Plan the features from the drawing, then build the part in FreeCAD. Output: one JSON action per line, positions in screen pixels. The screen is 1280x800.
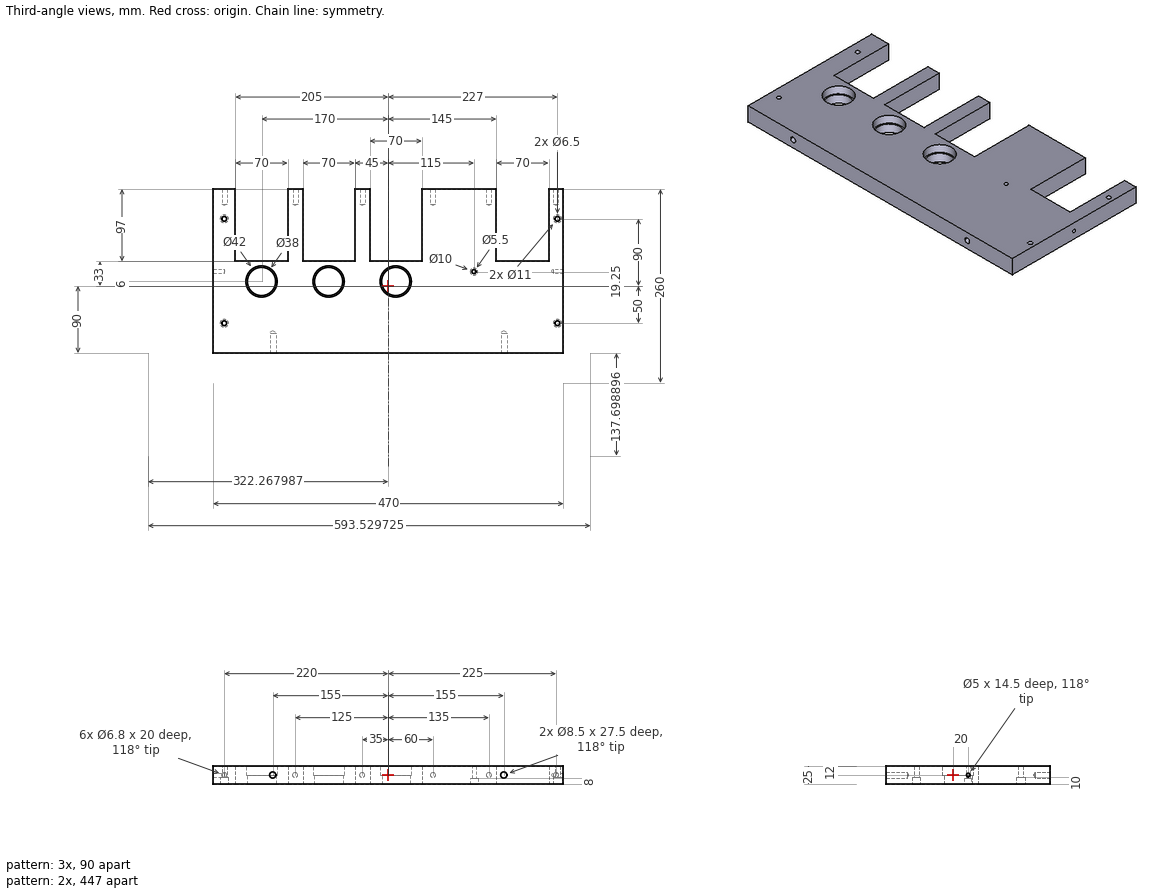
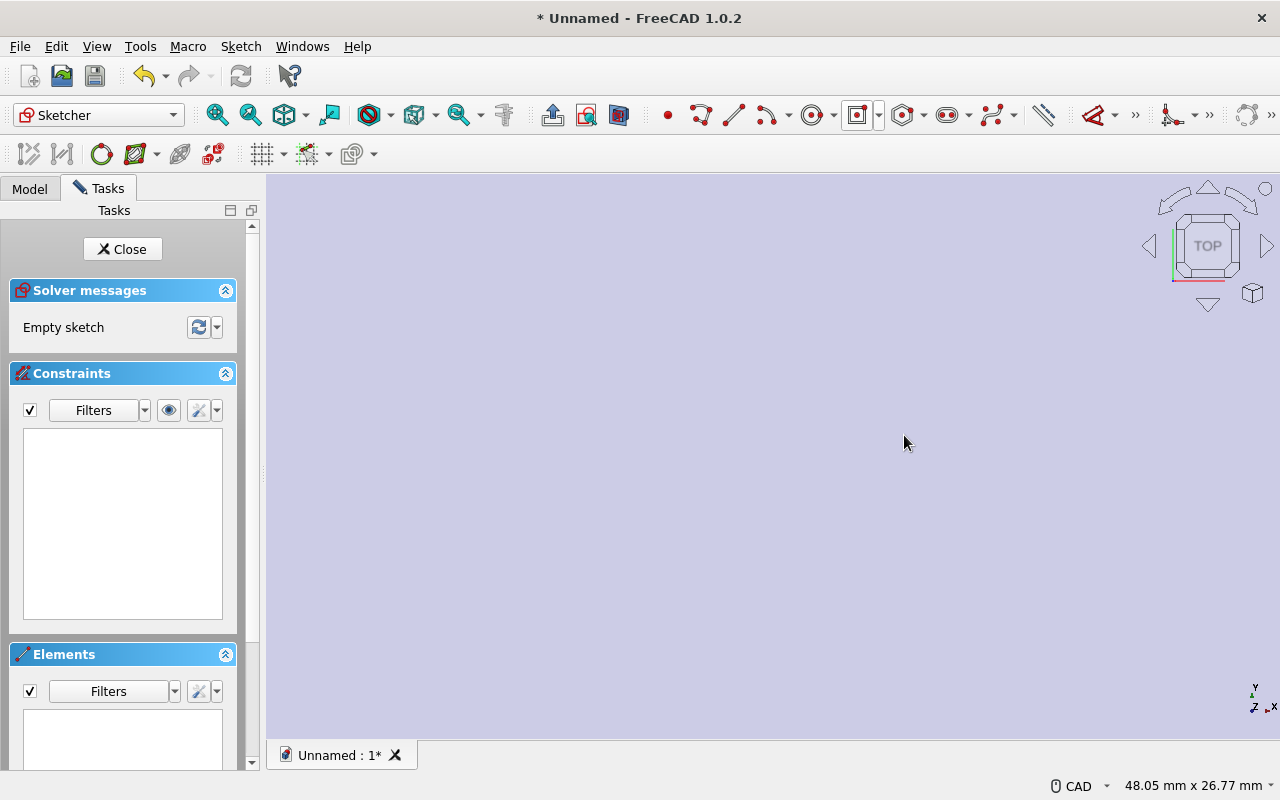
{"action": "scroll", "coordinate": [681, 450], "scroll_direction": "up", "scroll_amount": 6}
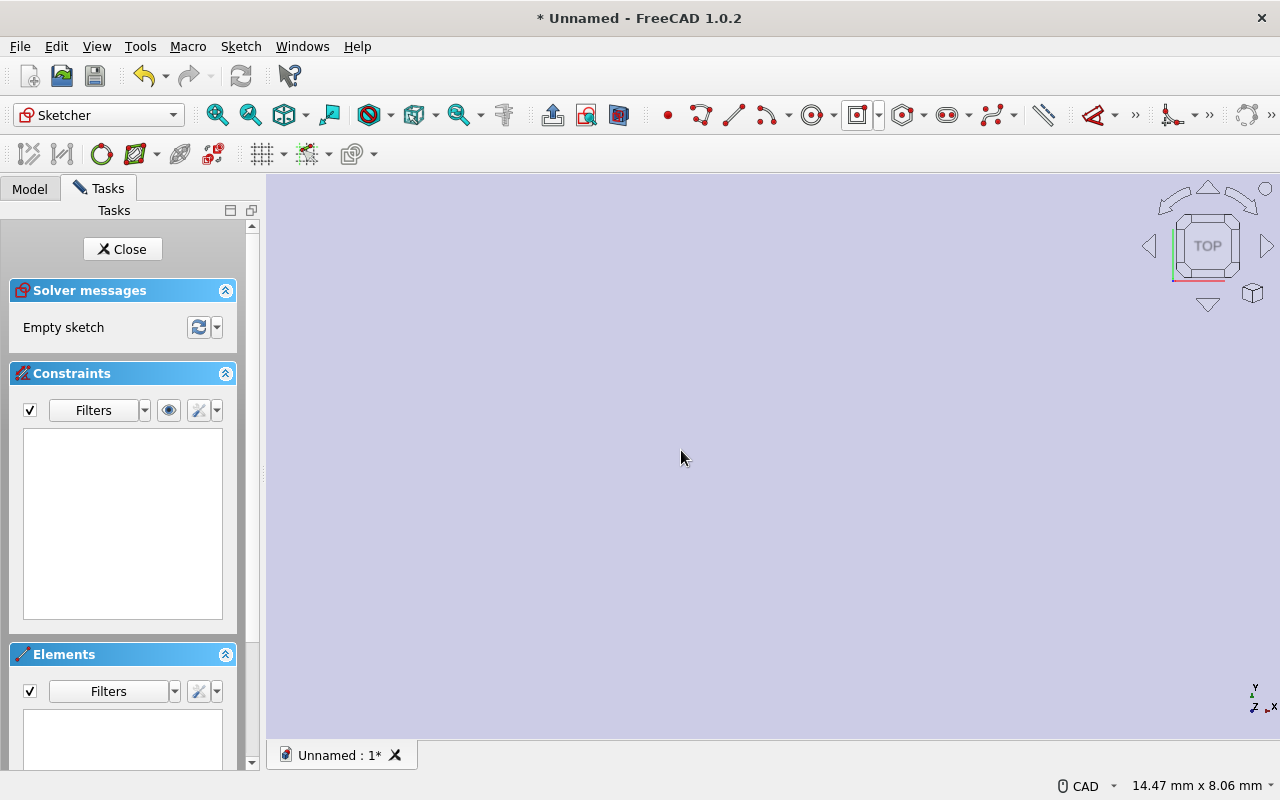
{"action": "left_click", "coordinate": [812, 116]}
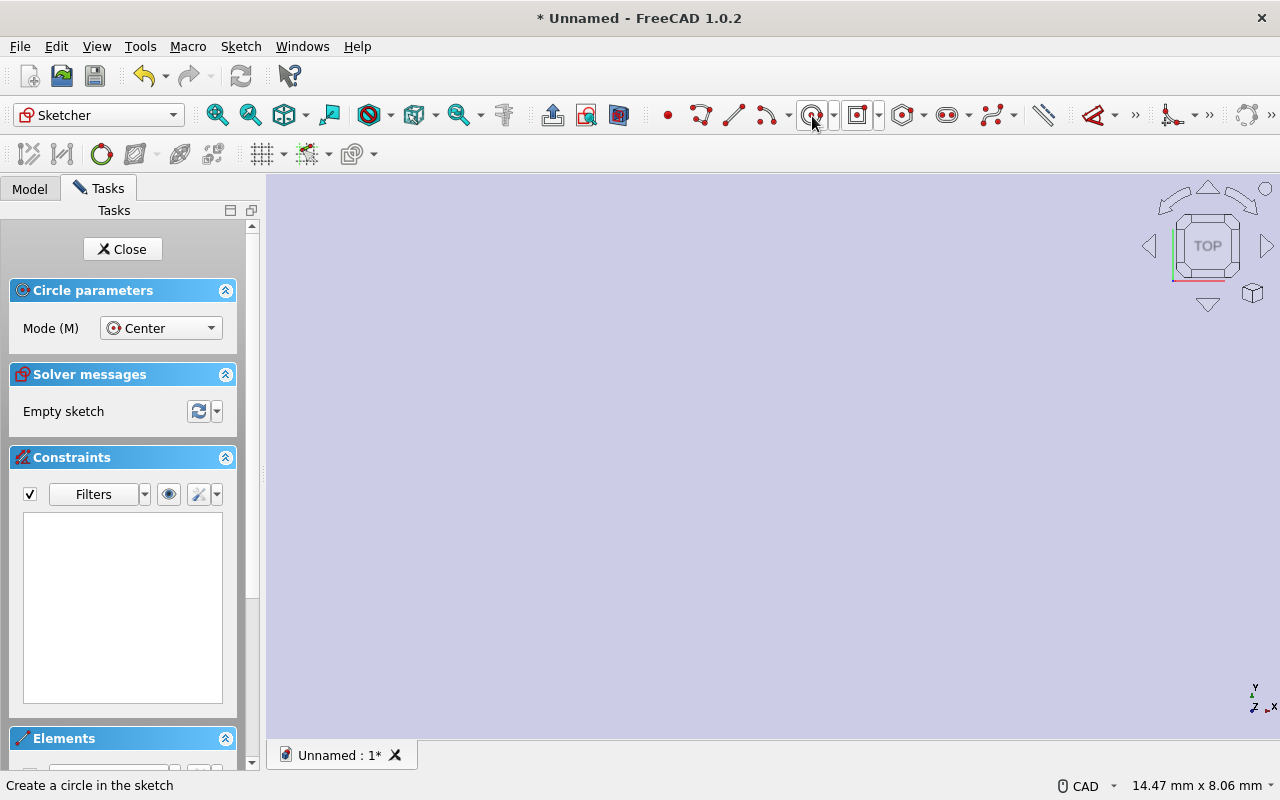
{"action": "left_click", "coordinate": [703, 455]}
{"action": "mouse_move", "coordinate": [839, 318]}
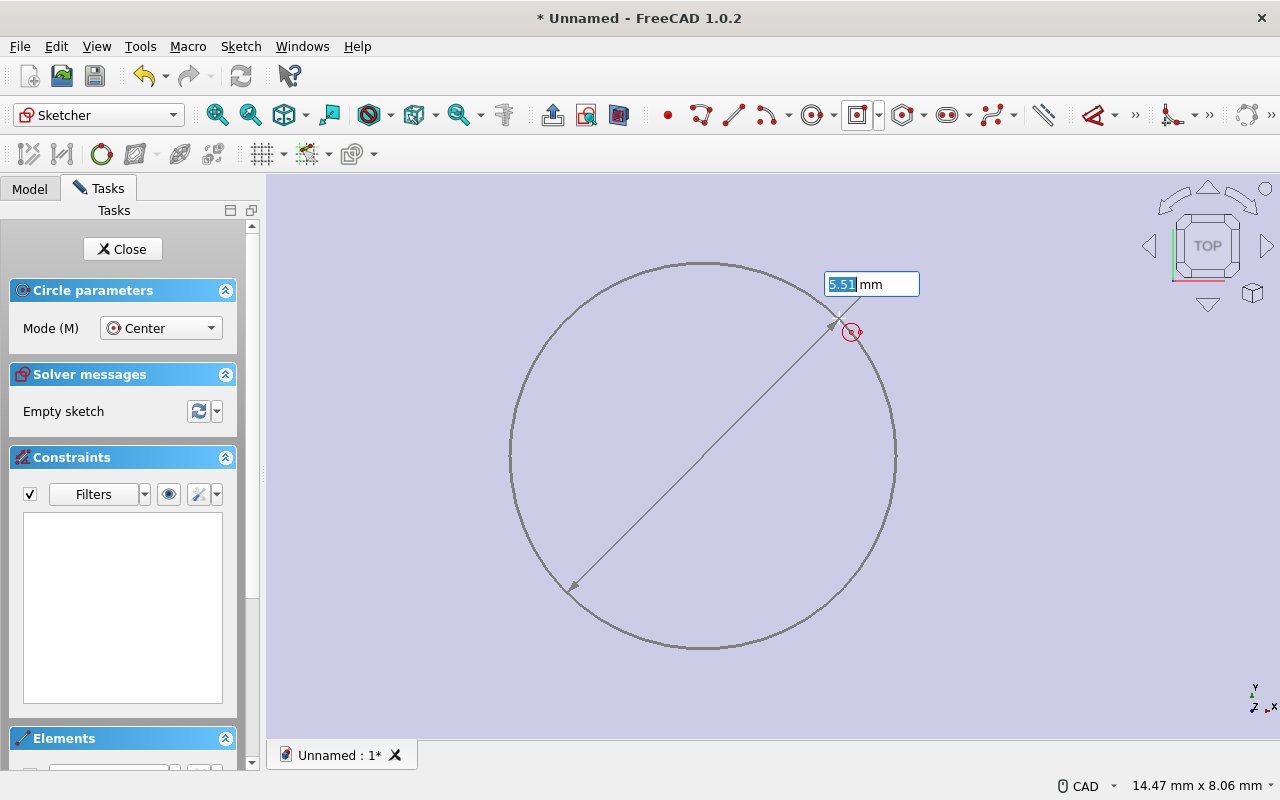
{"action": "type", "text": "5.5"}
{"action": "key", "text": "Return"}
{"action": "key", "text": "Escape"}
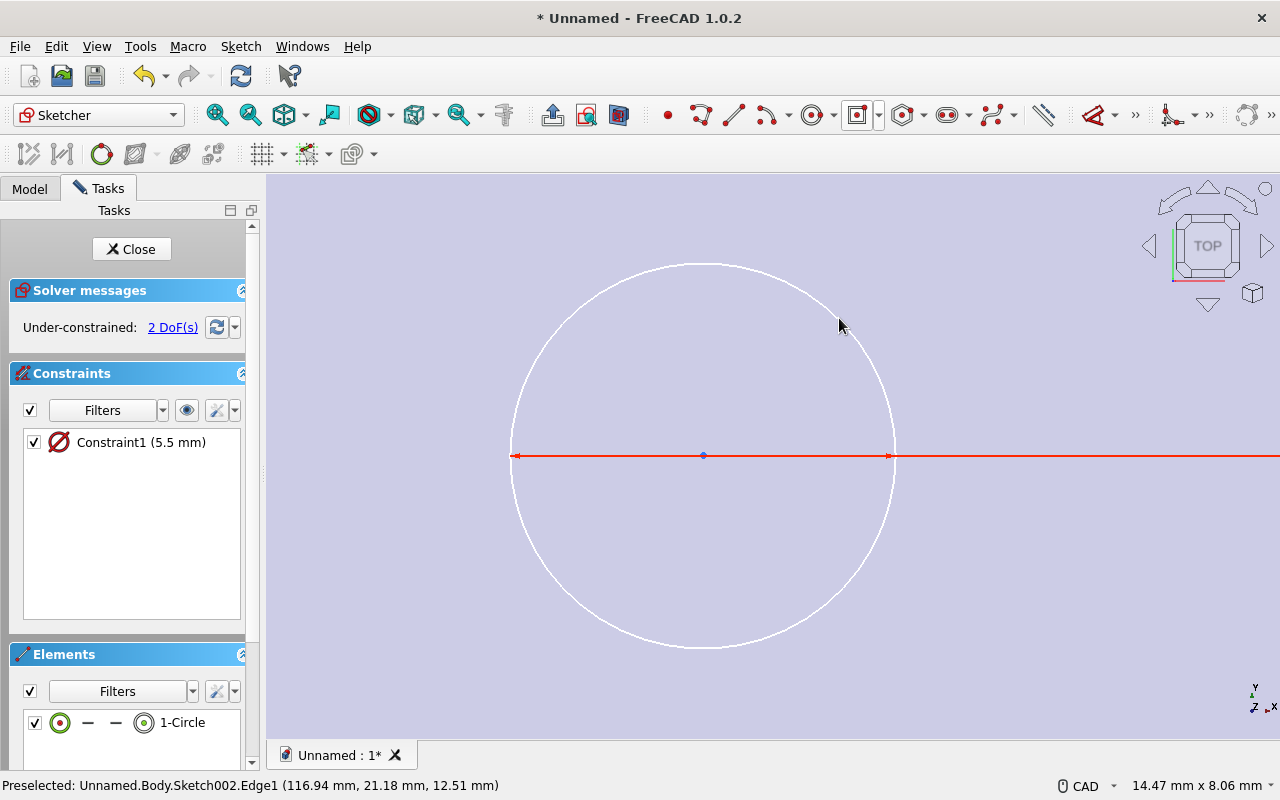
{"action": "left_click", "coordinate": [1092, 116]}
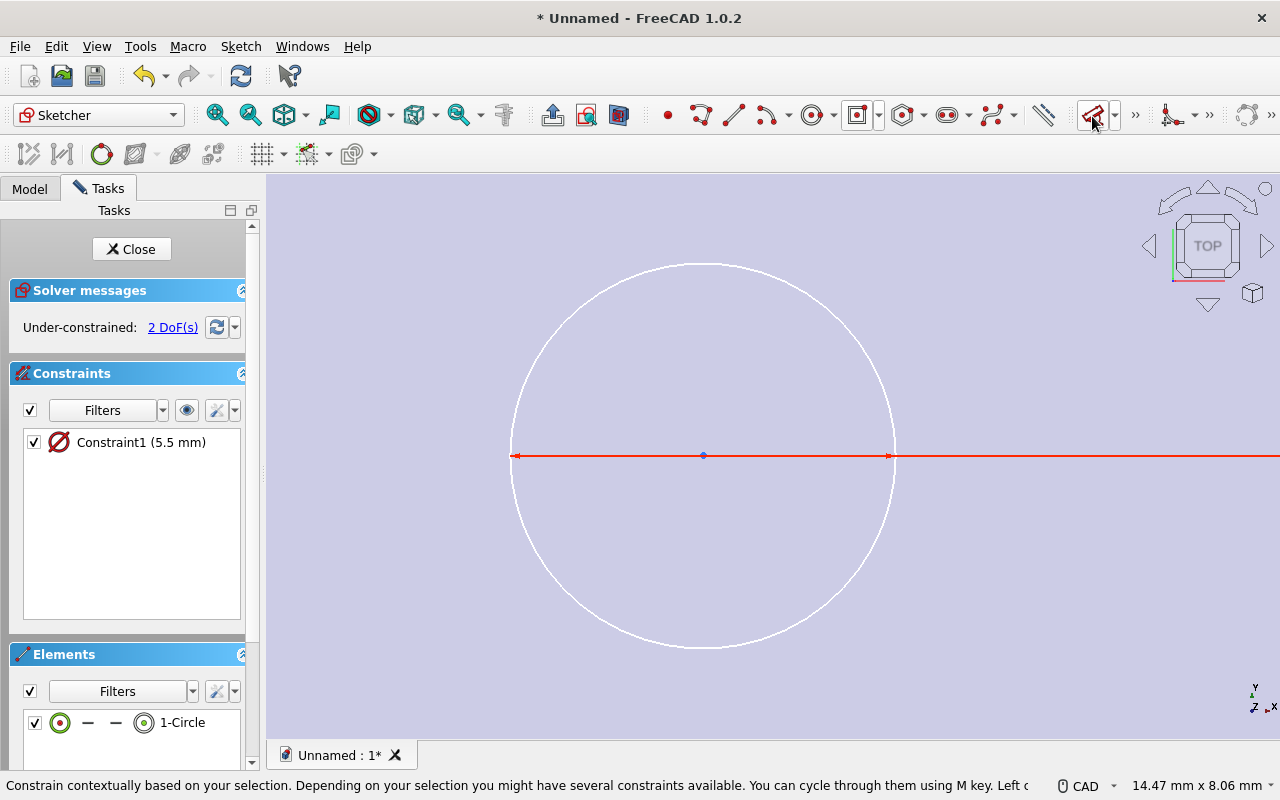
{"action": "left_click", "coordinate": [703, 456]}
{"action": "left_click", "coordinate": [498, 422]}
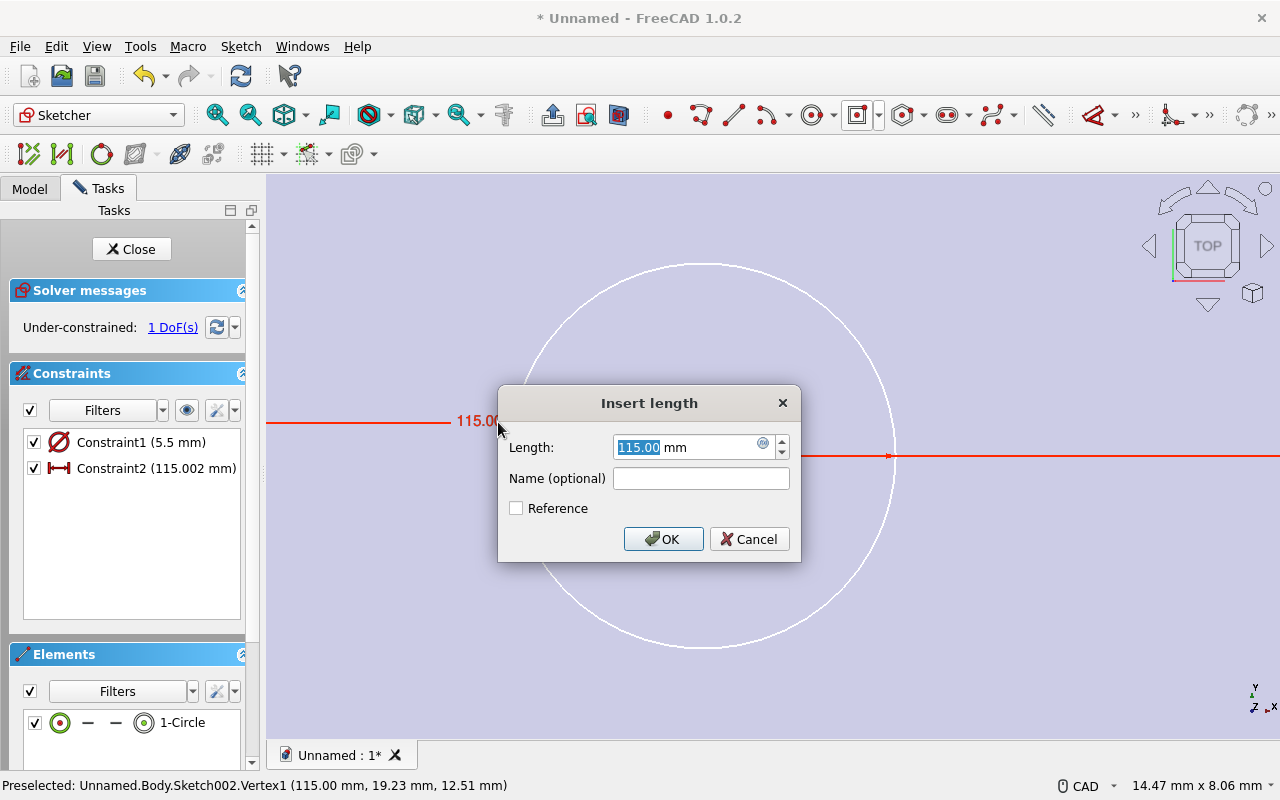
{"action": "type", "text": "115"}
{"action": "key", "text": "Return"}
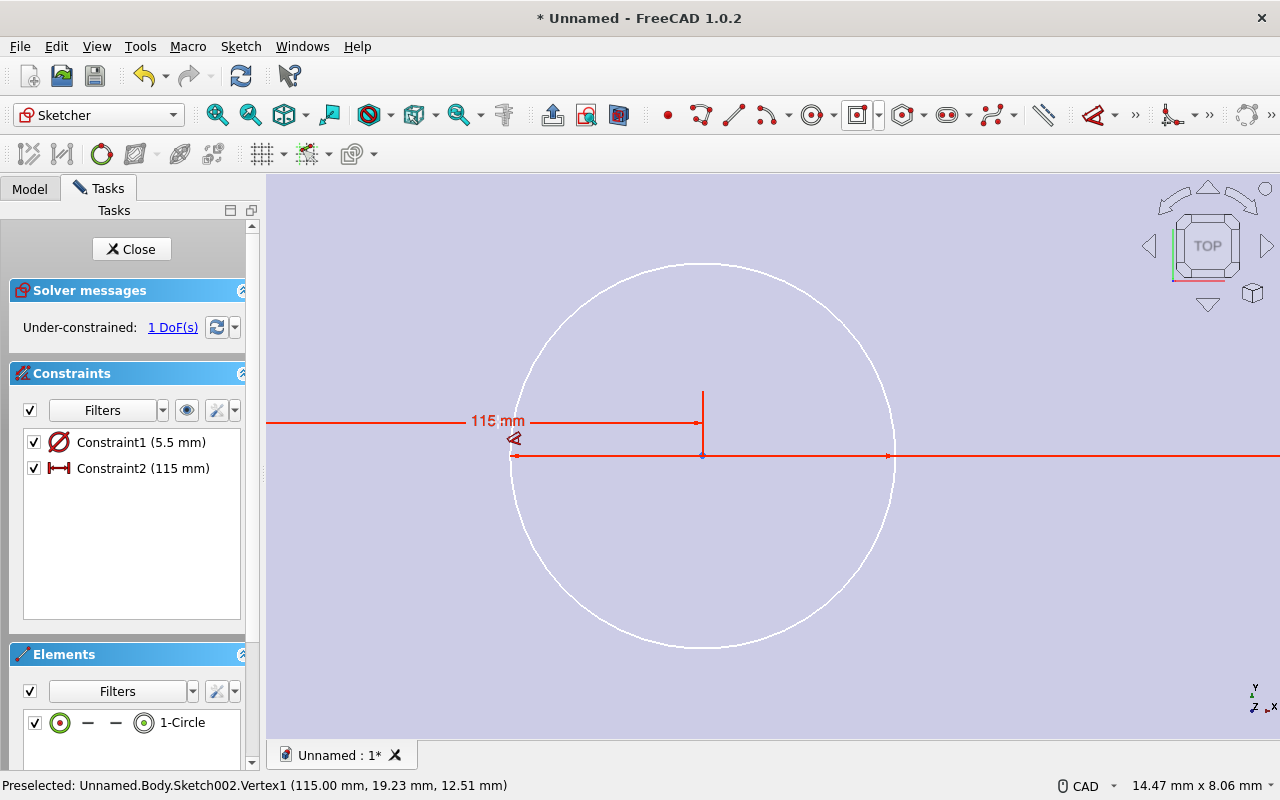
{"action": "left_click", "coordinate": [703, 456]}
{"action": "left_click", "coordinate": [737, 584]}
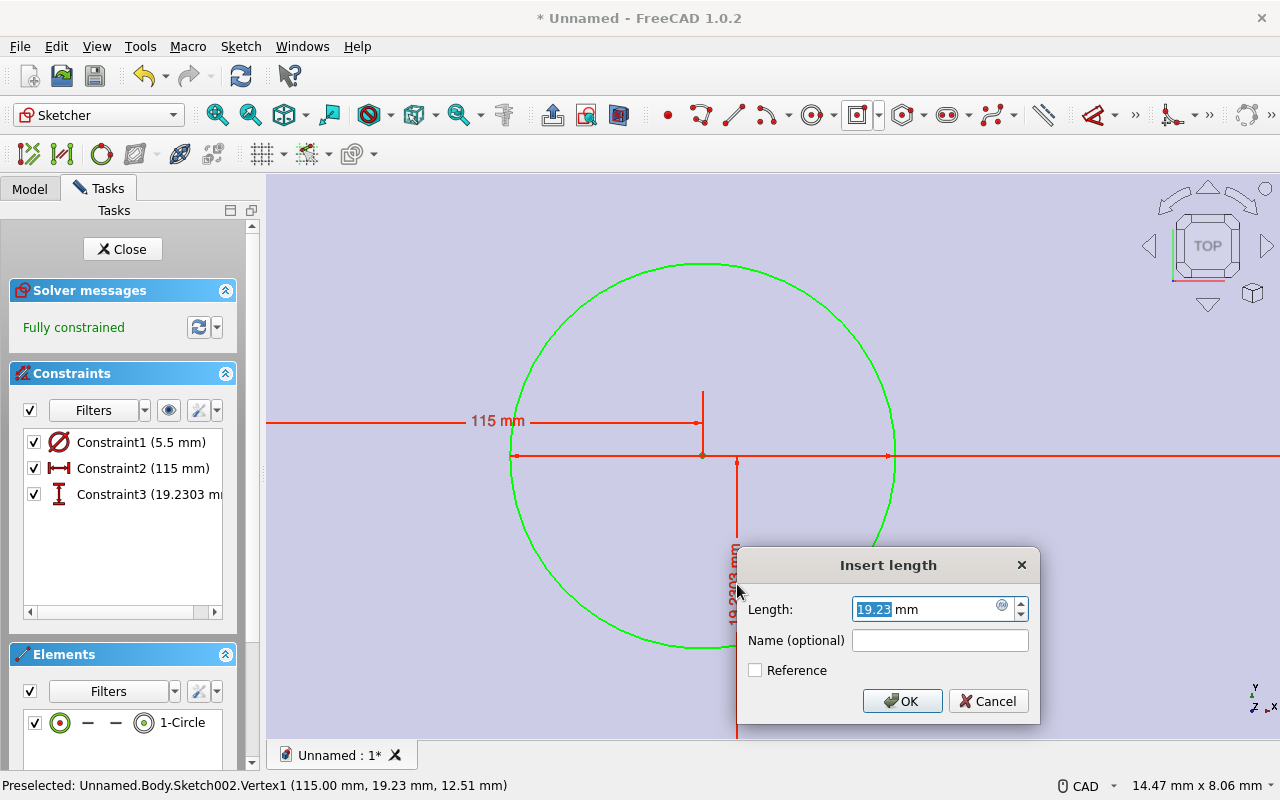
{"action": "type", "text": "19.25"}
{"action": "key", "text": "Return"}
{"action": "key", "text": "Escape"}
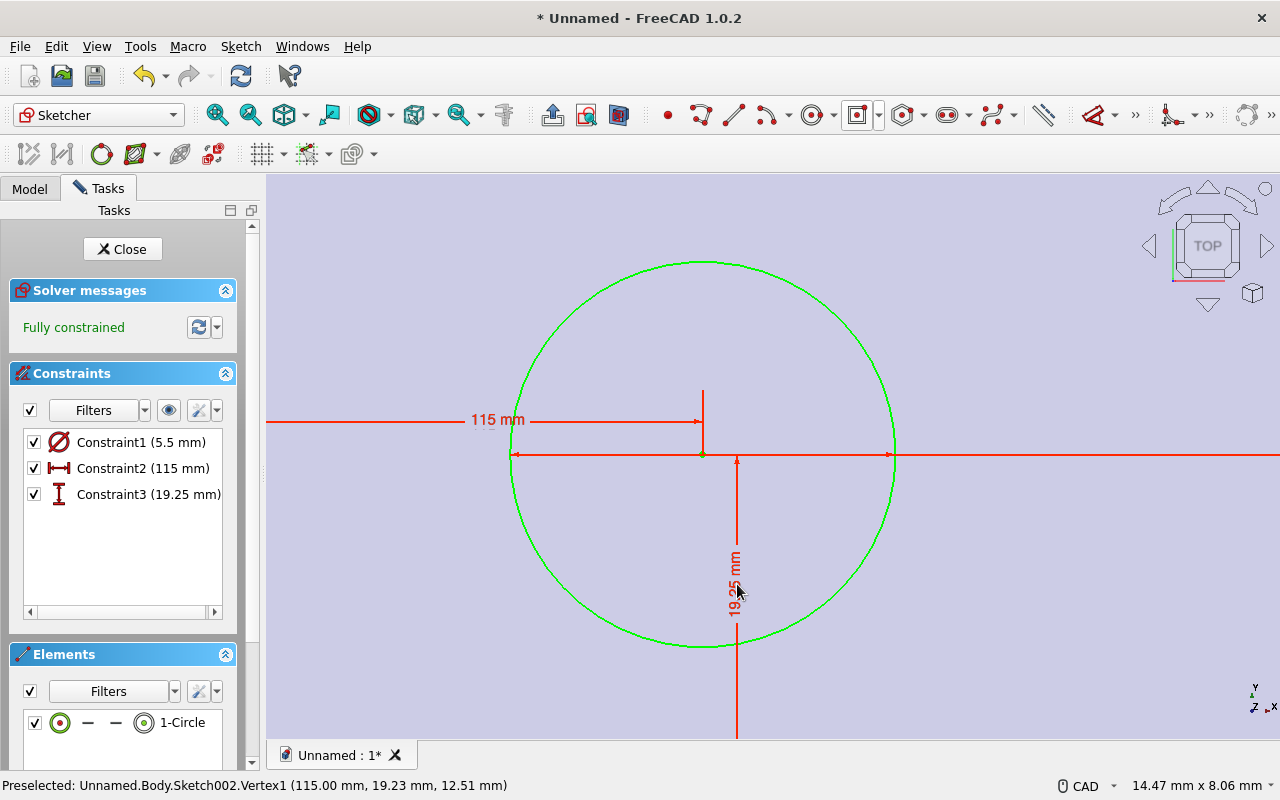
{"action": "left_click", "coordinate": [123, 249]}